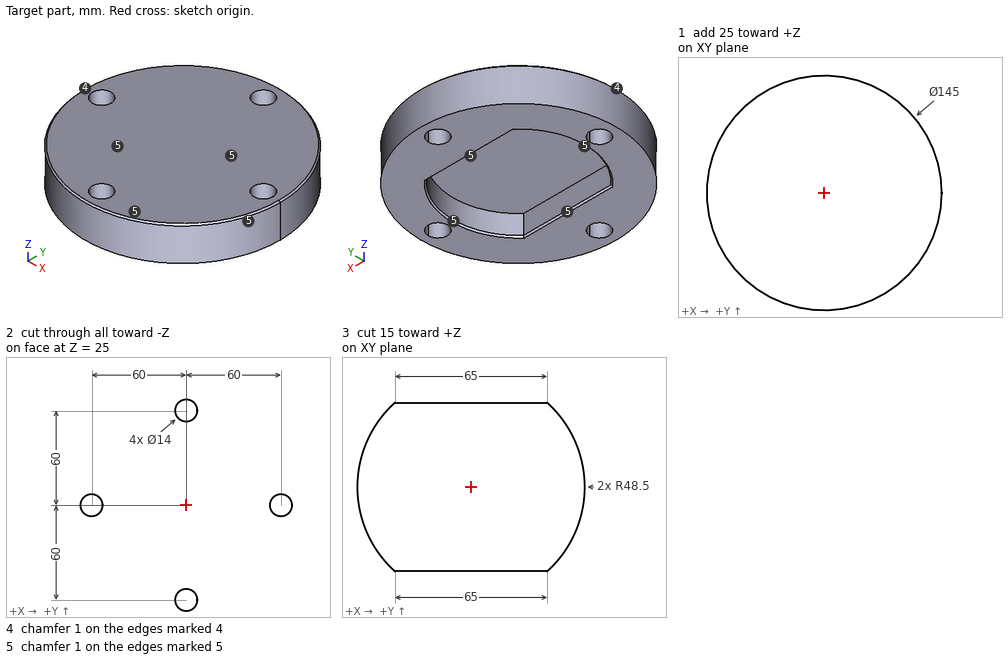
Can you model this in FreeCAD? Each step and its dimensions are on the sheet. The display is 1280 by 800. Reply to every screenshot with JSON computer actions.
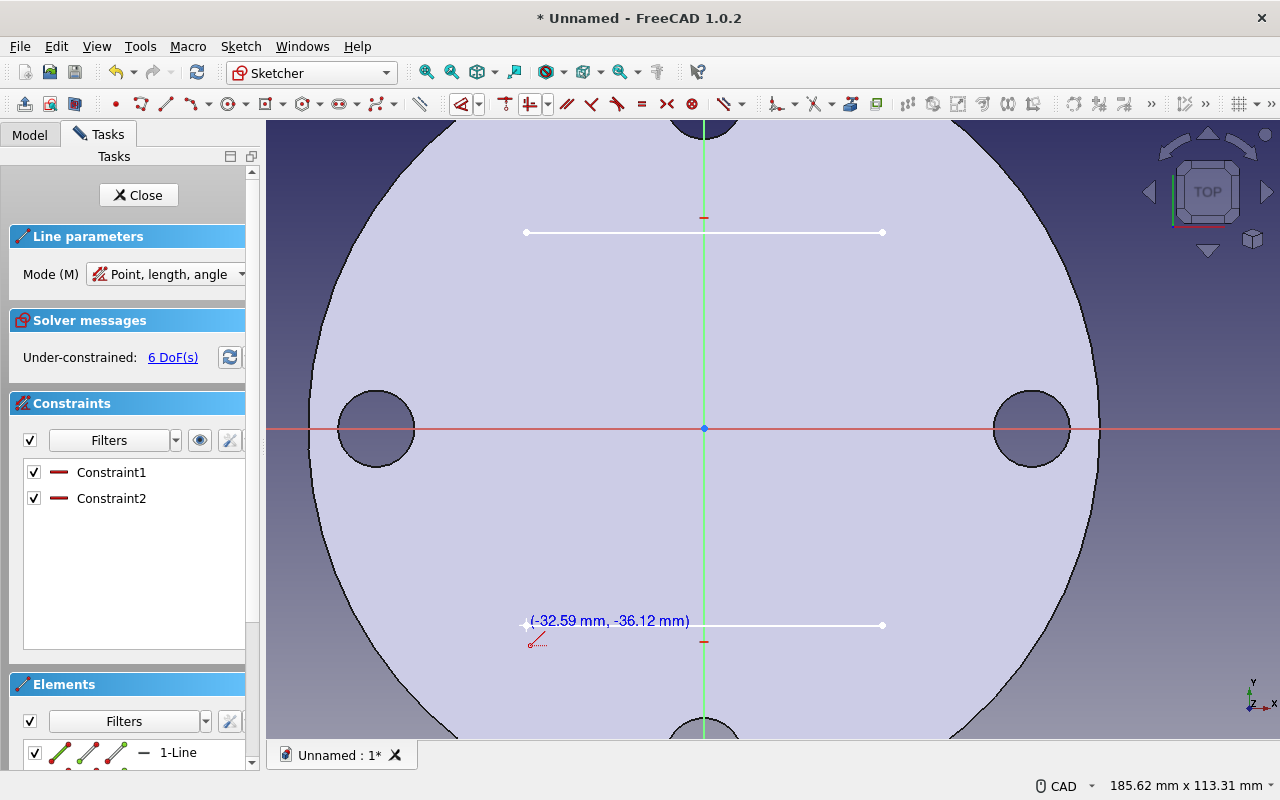
{"action": "left_click", "coordinate": [190, 104]}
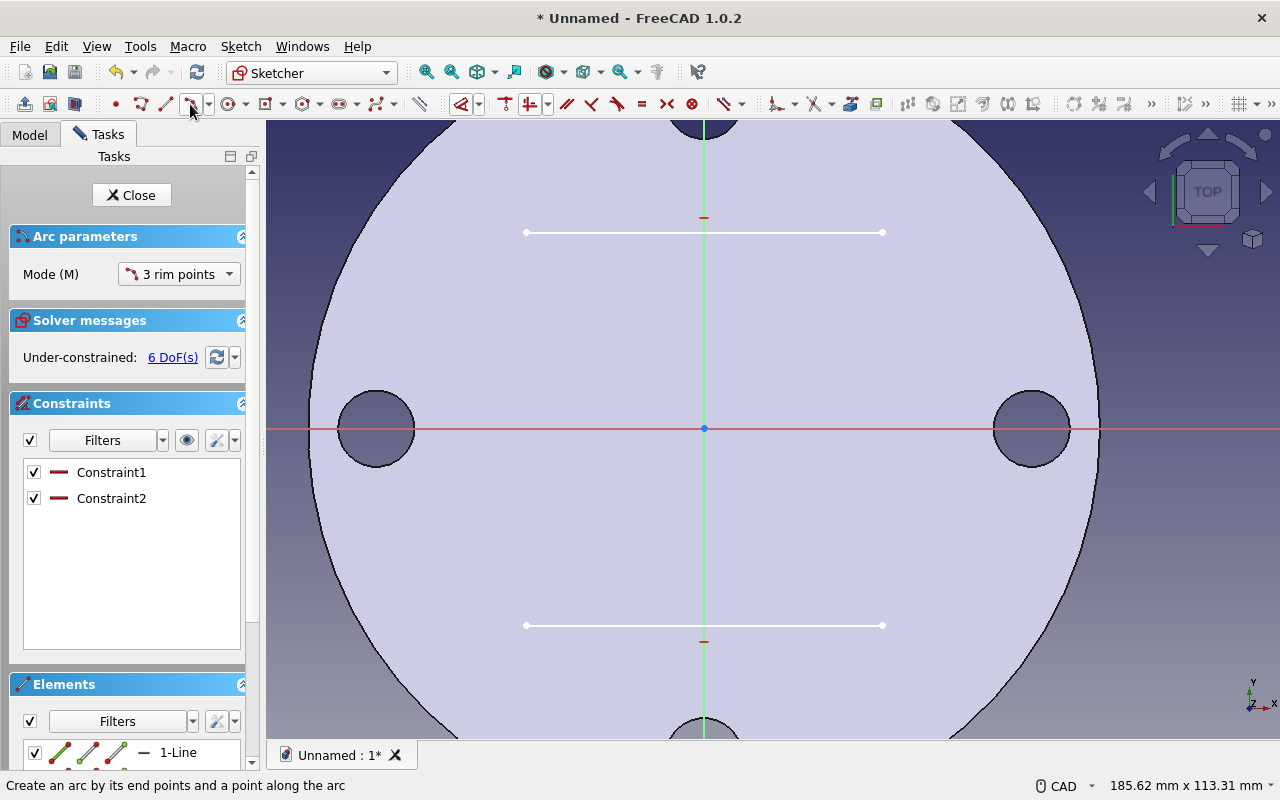
{"action": "left_click", "coordinate": [882, 233]}
{"action": "left_click", "coordinate": [882, 626]}
{"action": "left_click", "coordinate": [965, 473]}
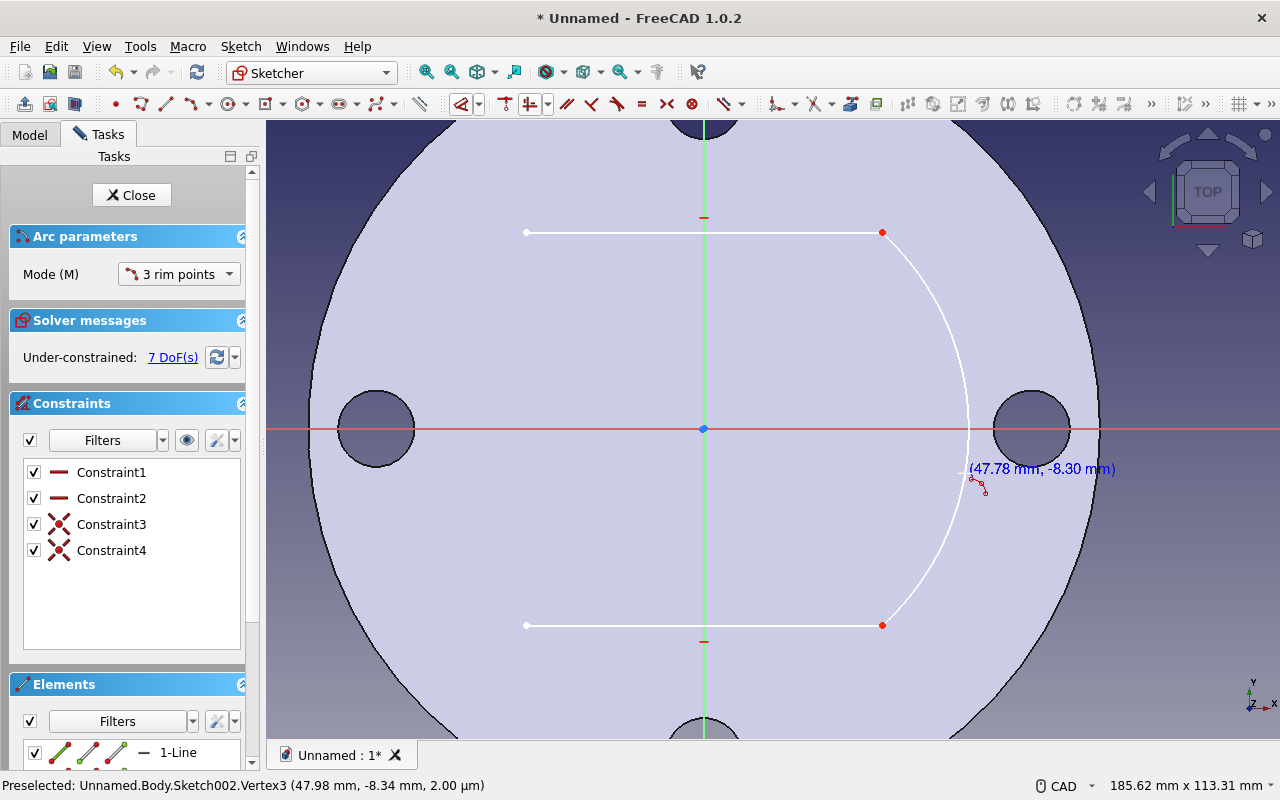
{"action": "left_click", "coordinate": [526, 626]}
{"action": "left_click", "coordinate": [526, 233]}
{"action": "left_click", "coordinate": [443, 385]}
{"action": "key", "text": "Escape"}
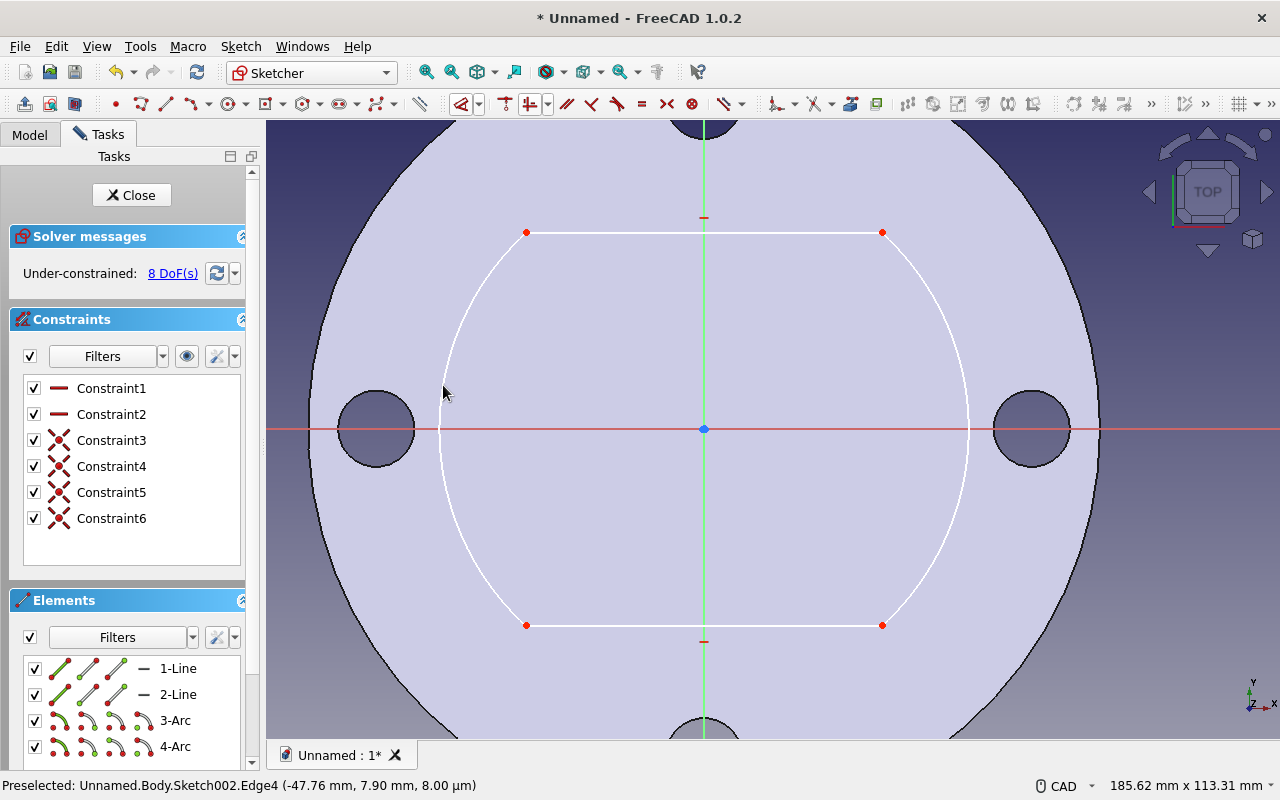
{"action": "left_click", "coordinate": [954, 516]}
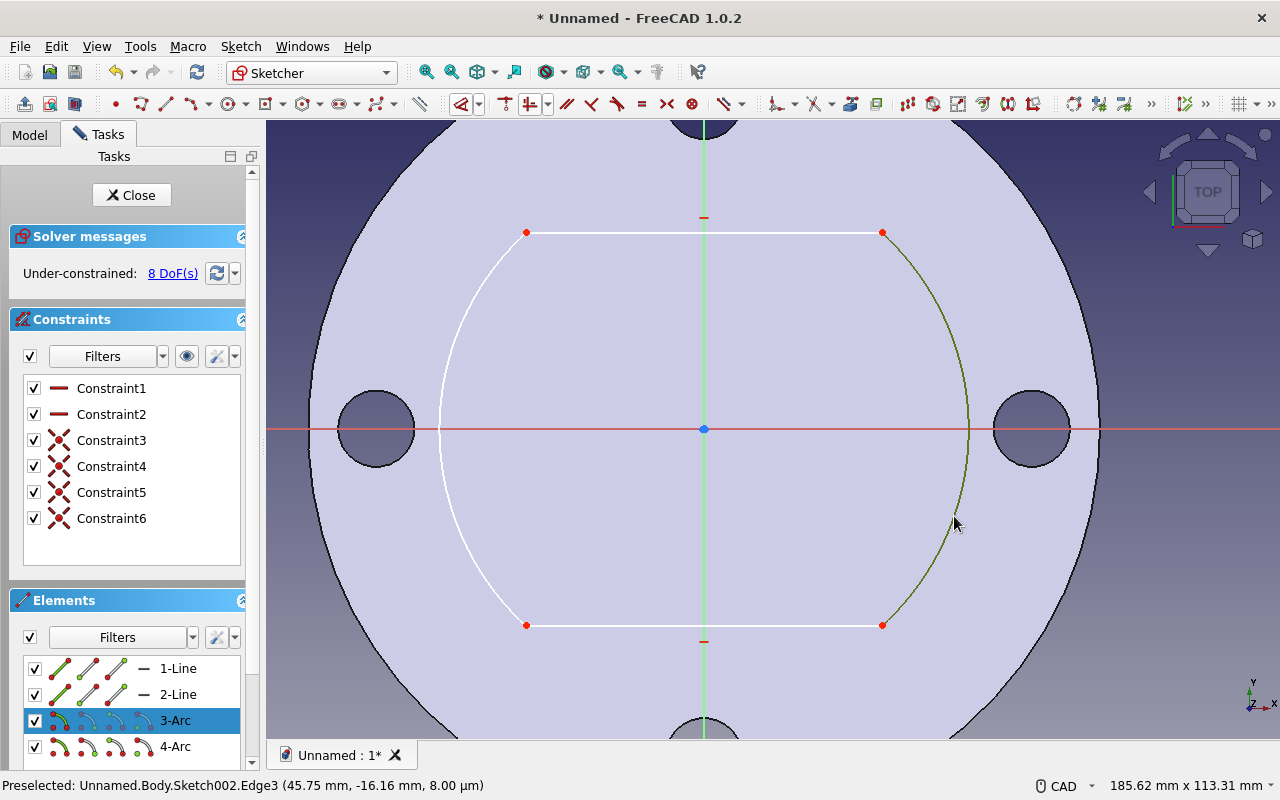
{"action": "left_click", "coordinate": [454, 343]}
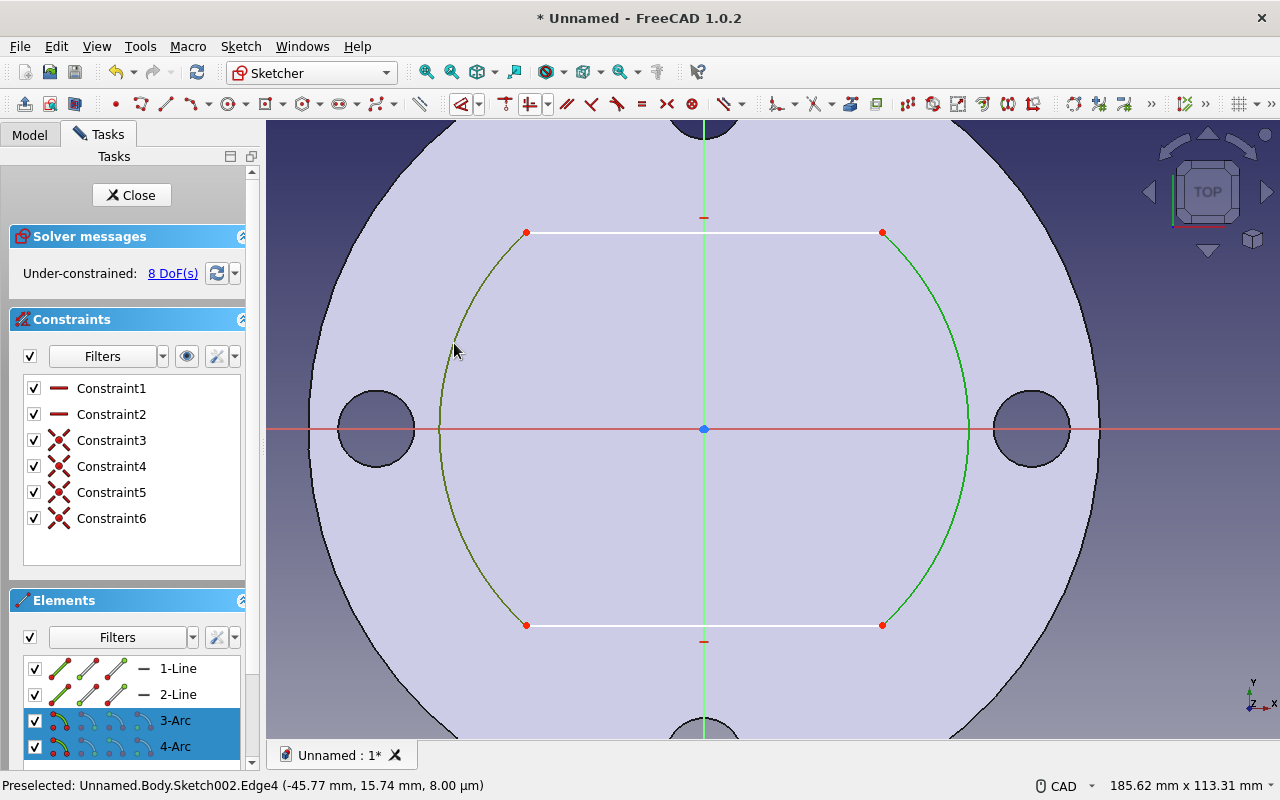
{"action": "left_click", "coordinate": [505, 104]}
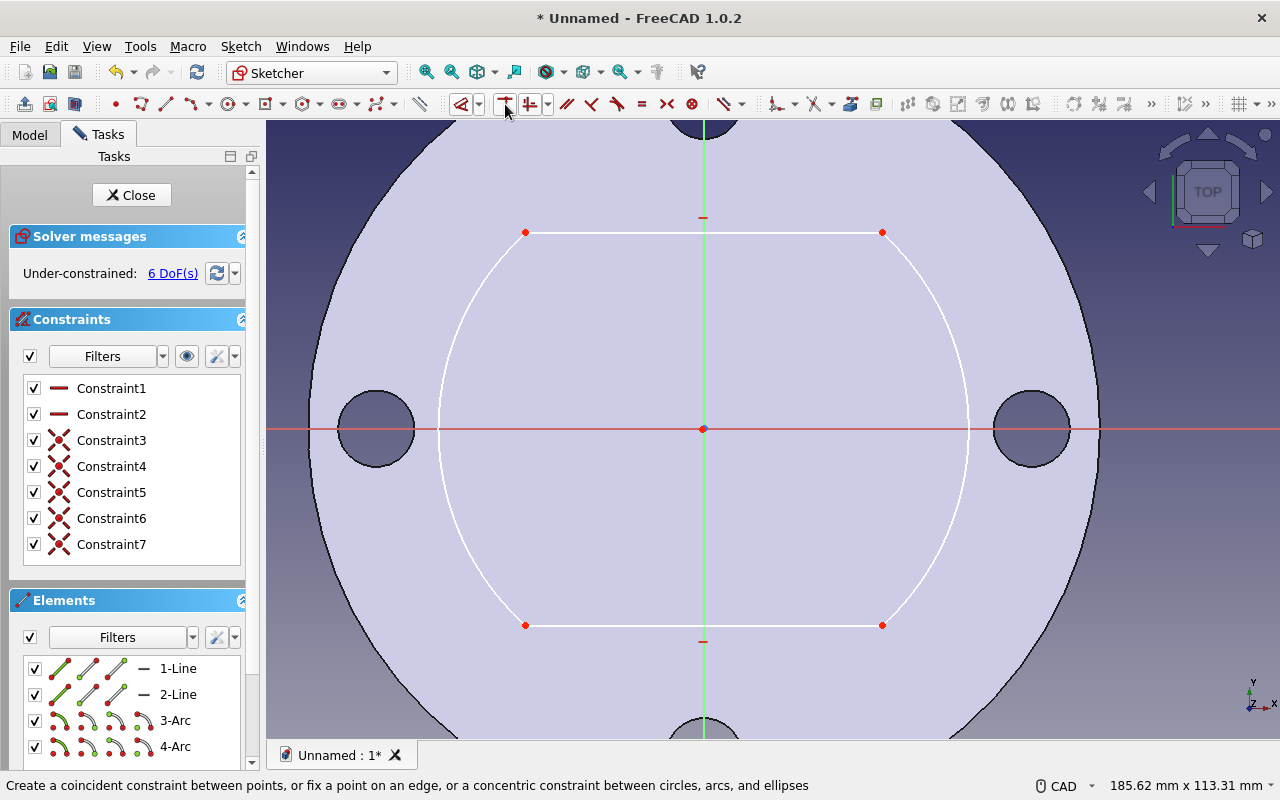
{"action": "left_click_drag", "start_coordinate": [693, 419], "coordinate": [714, 439]}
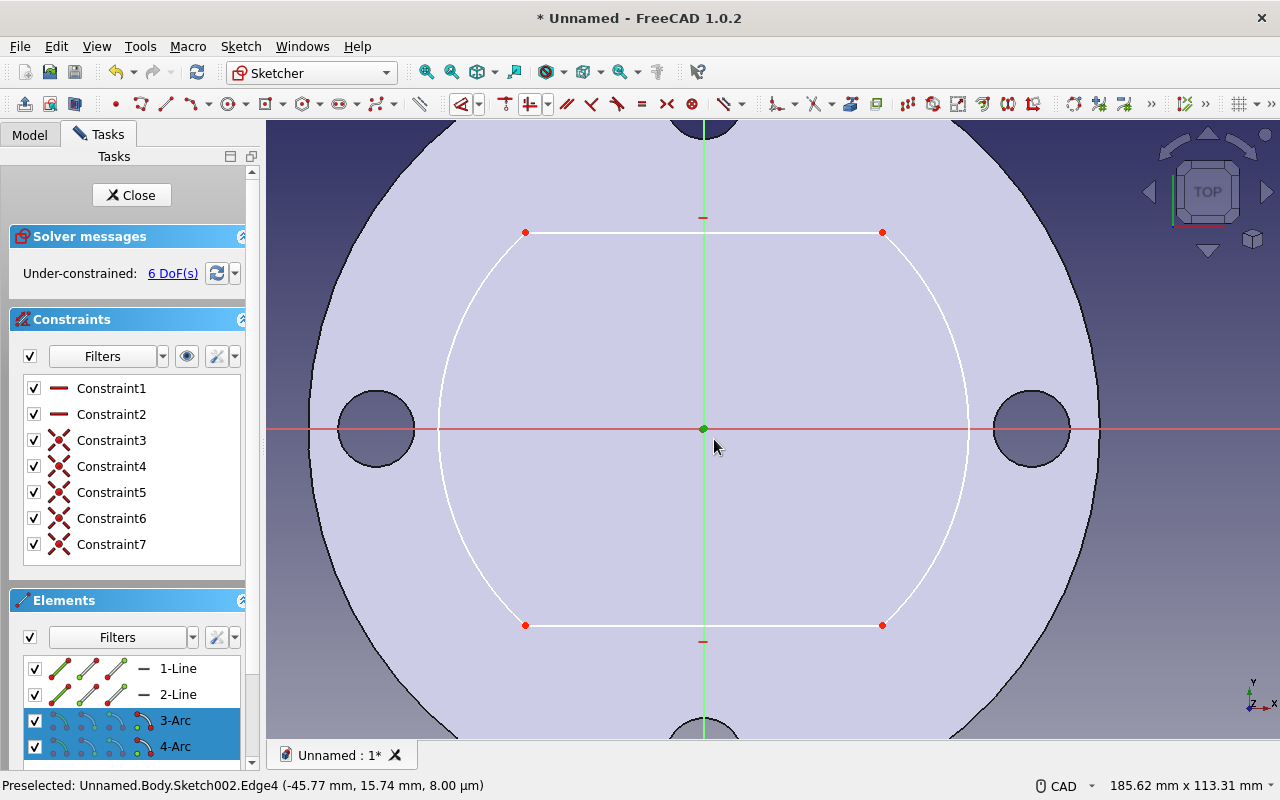
{"action": "left_click", "coordinate": [505, 104]}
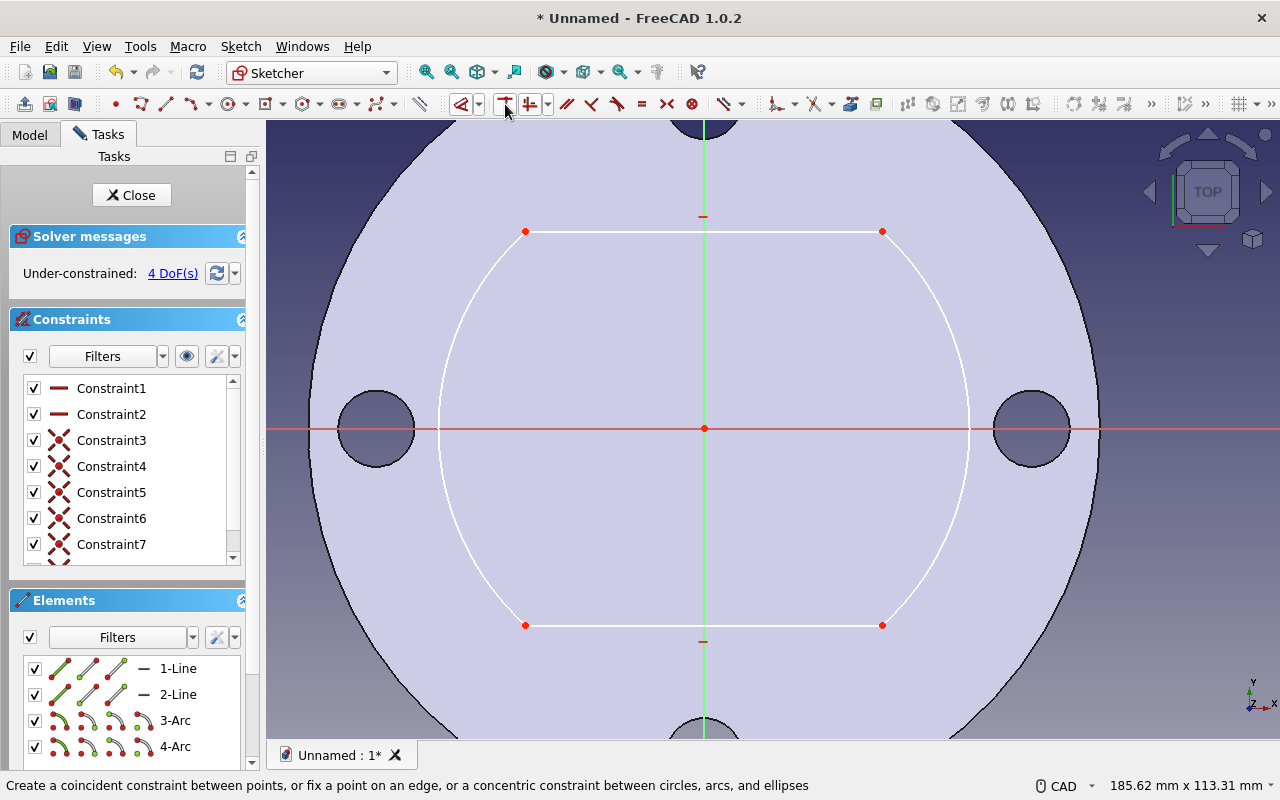
{"action": "left_click", "coordinate": [955, 516]}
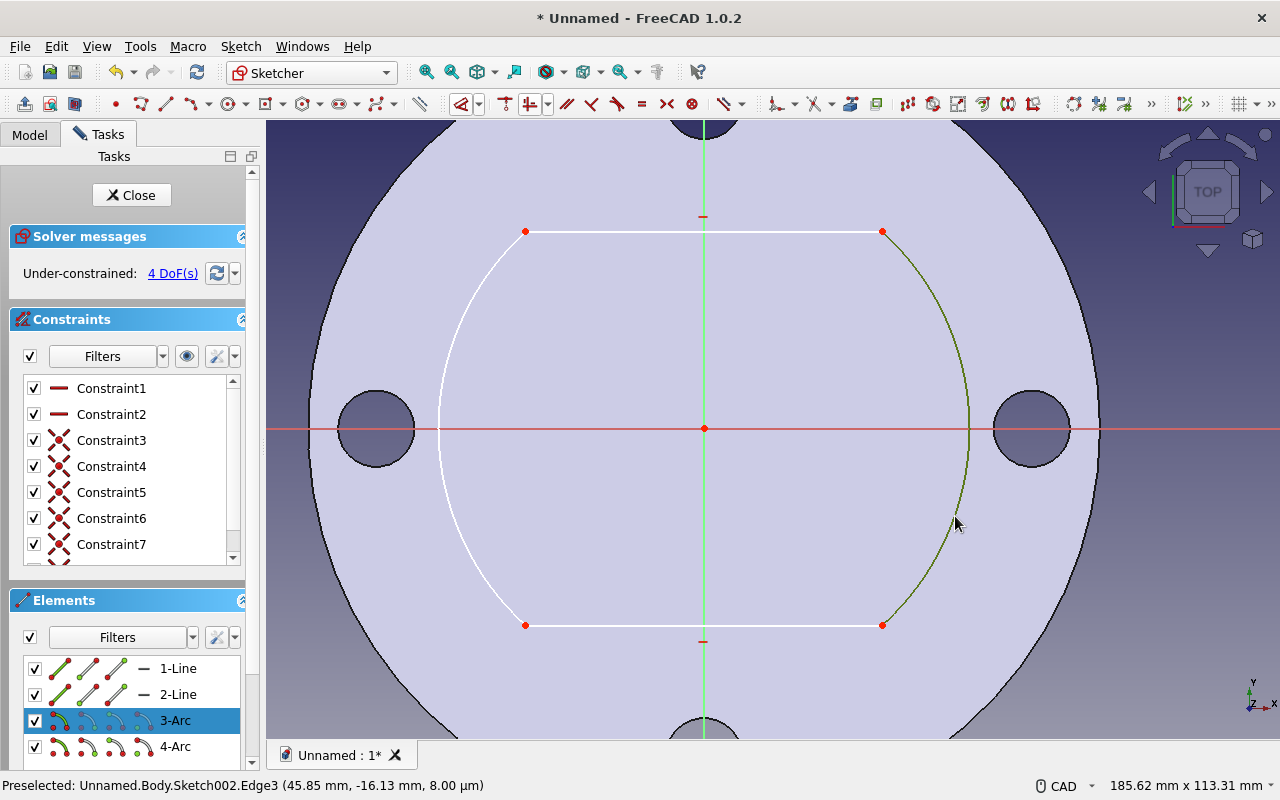
{"action": "left_click", "coordinate": [453, 342]}